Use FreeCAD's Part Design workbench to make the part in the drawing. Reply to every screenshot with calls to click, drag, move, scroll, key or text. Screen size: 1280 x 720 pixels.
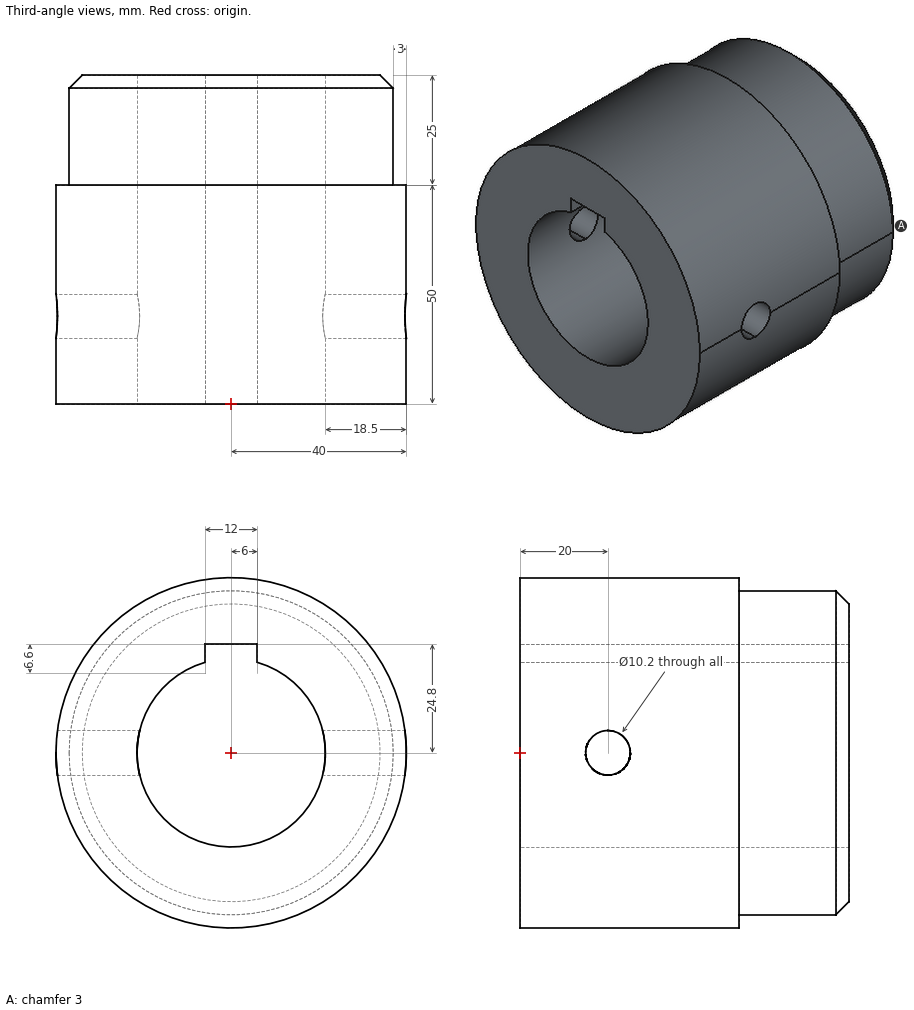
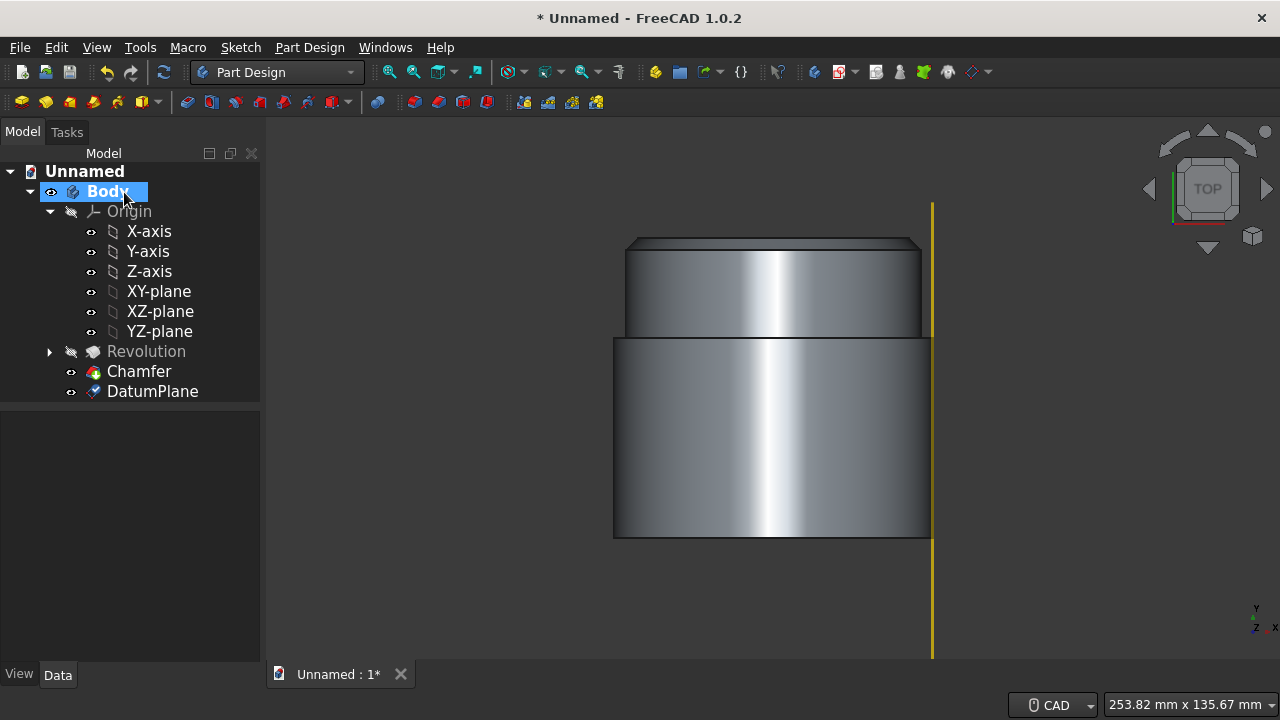
click(116, 392)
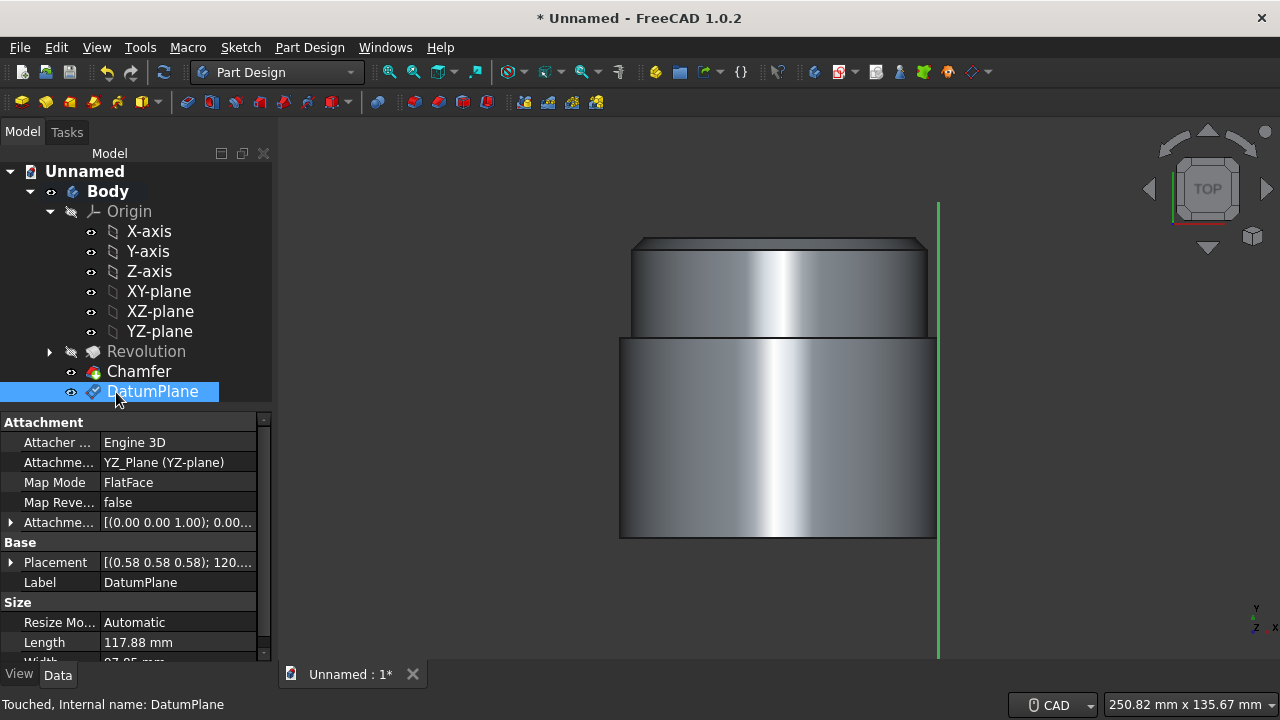
click(840, 72)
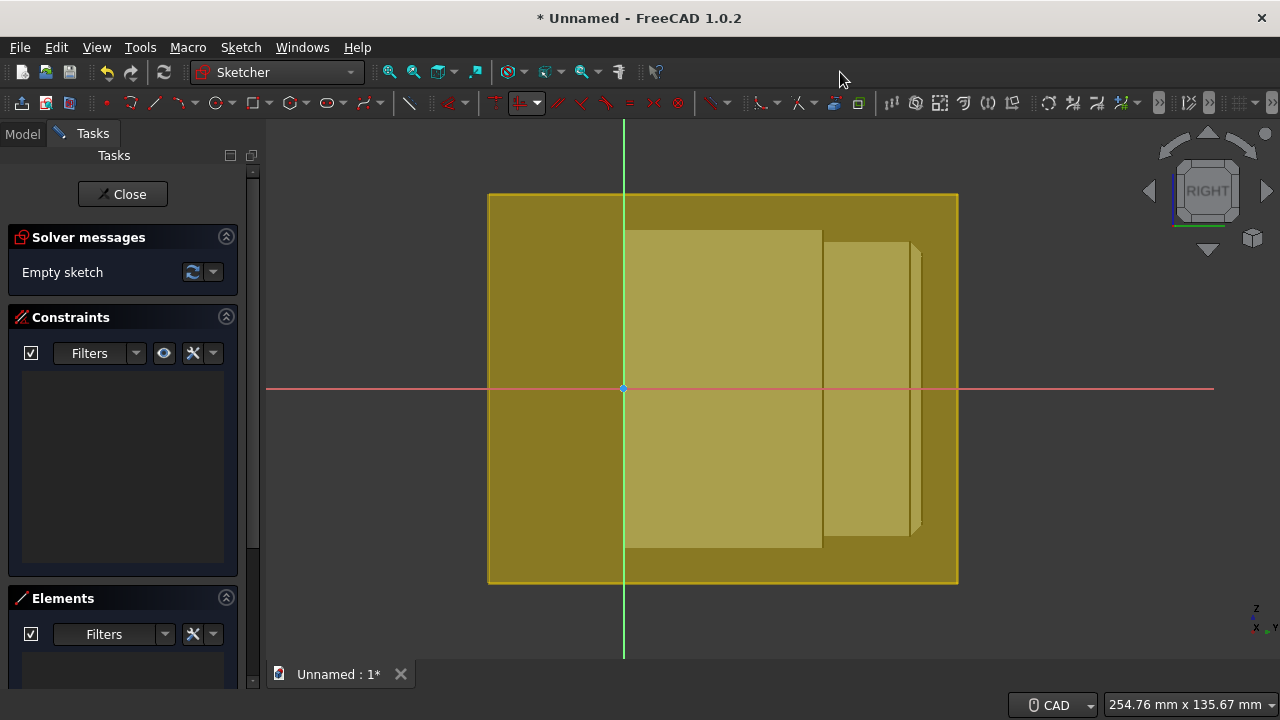
scroll(668, 389, up, 9)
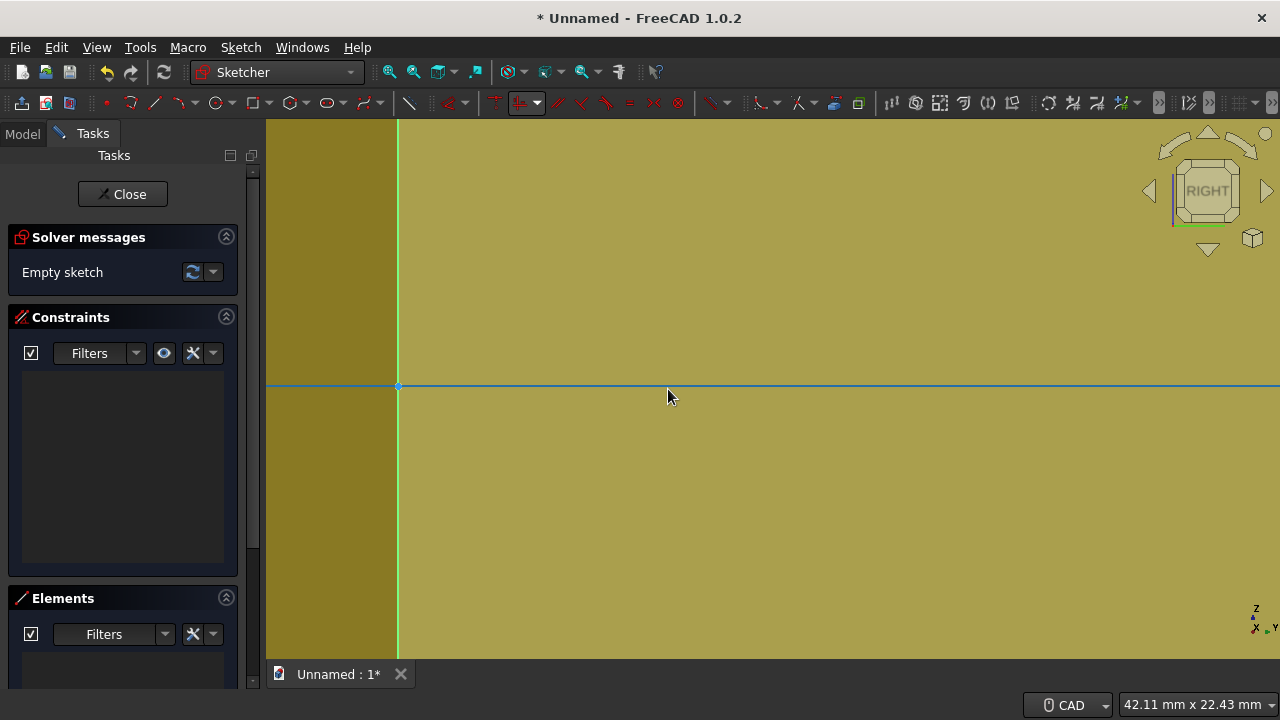
key(g)
key(c)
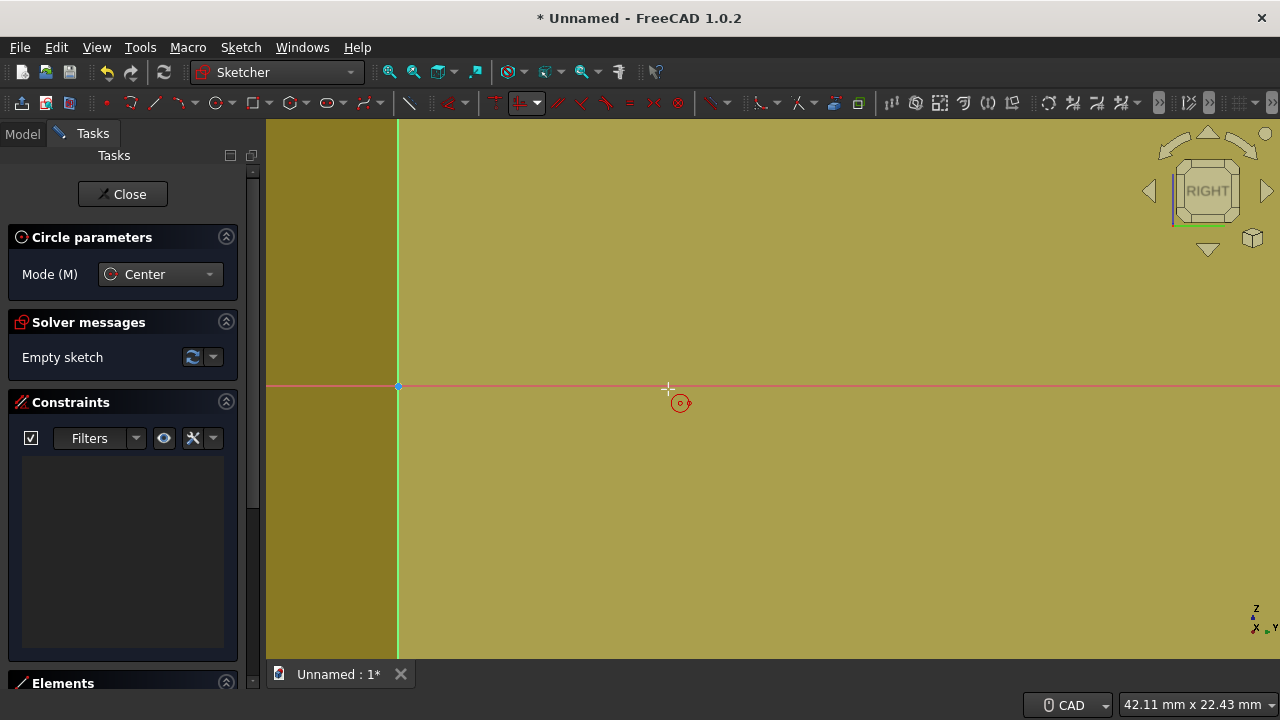
click(880, 386)
move(967, 300)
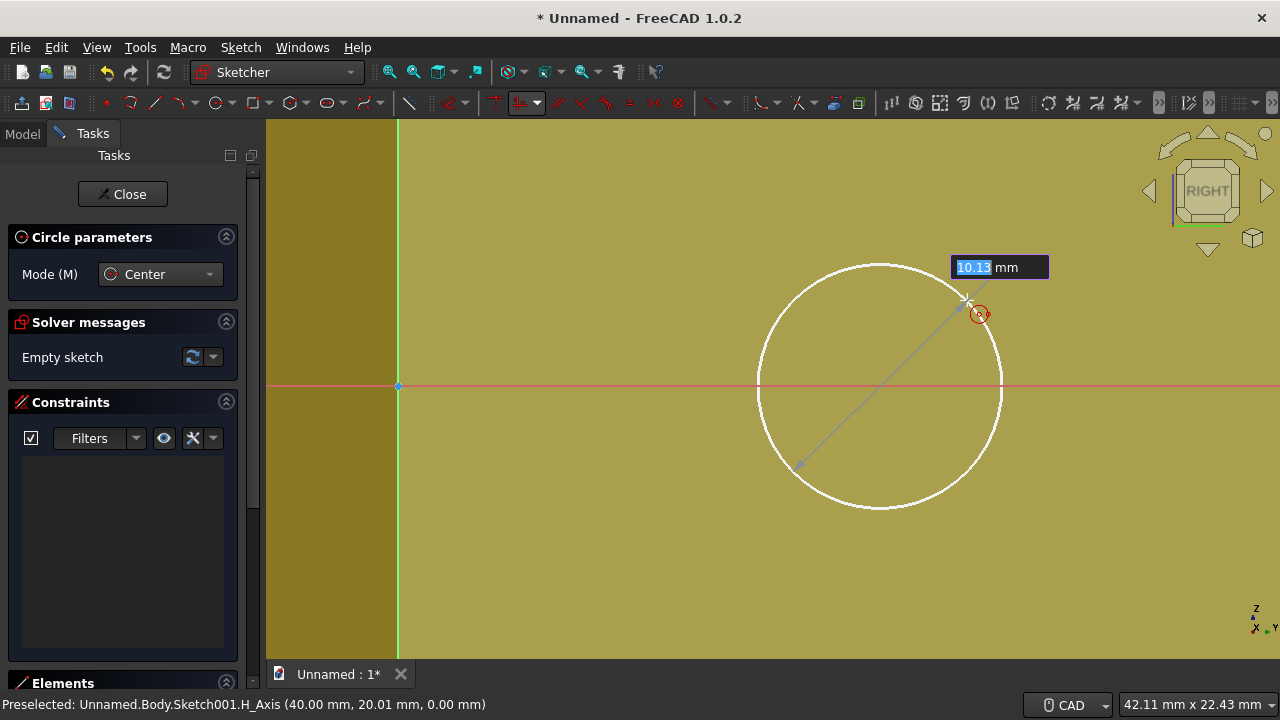
text(10.2)
key(Return)
key(Escape)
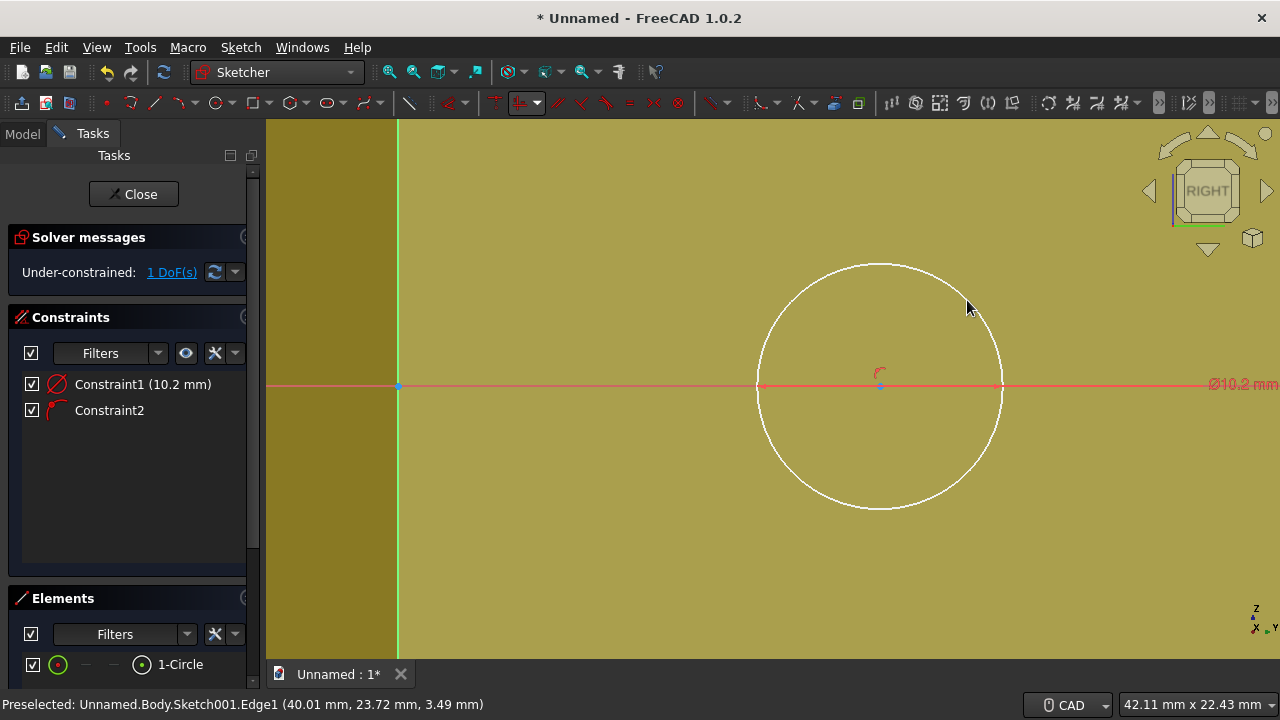
click(448, 104)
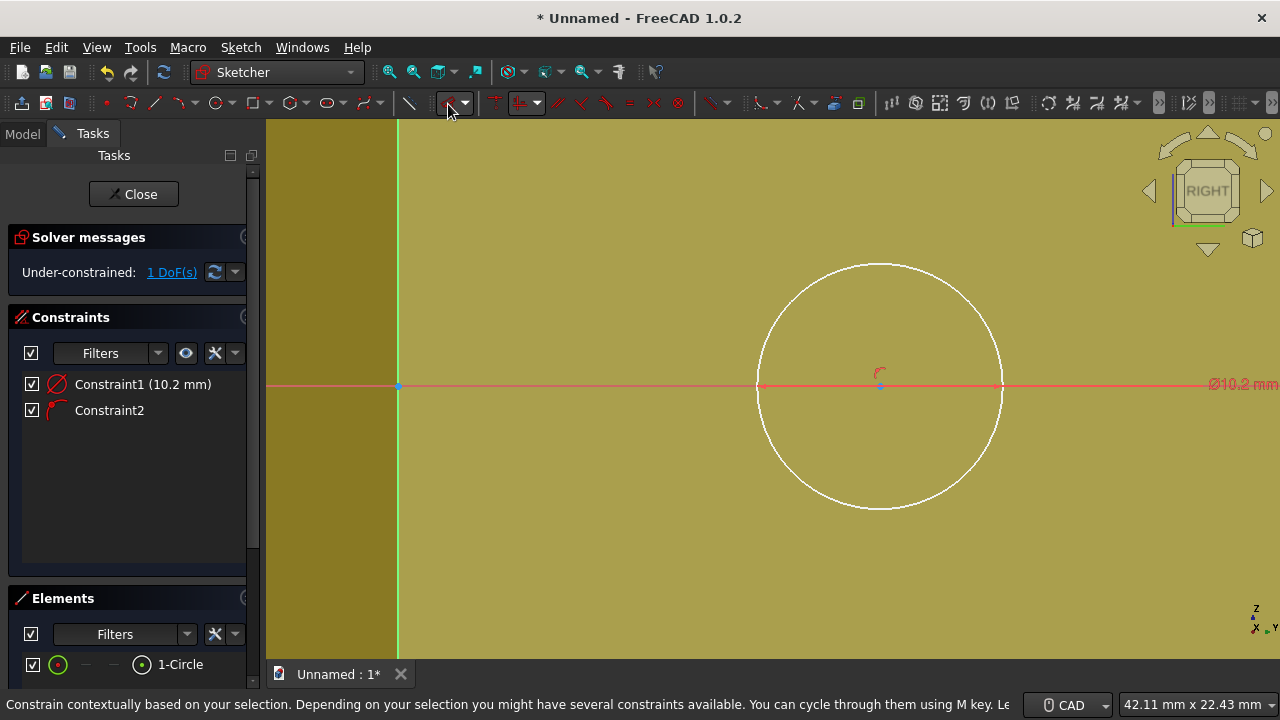
click(880, 386)
click(639, 420)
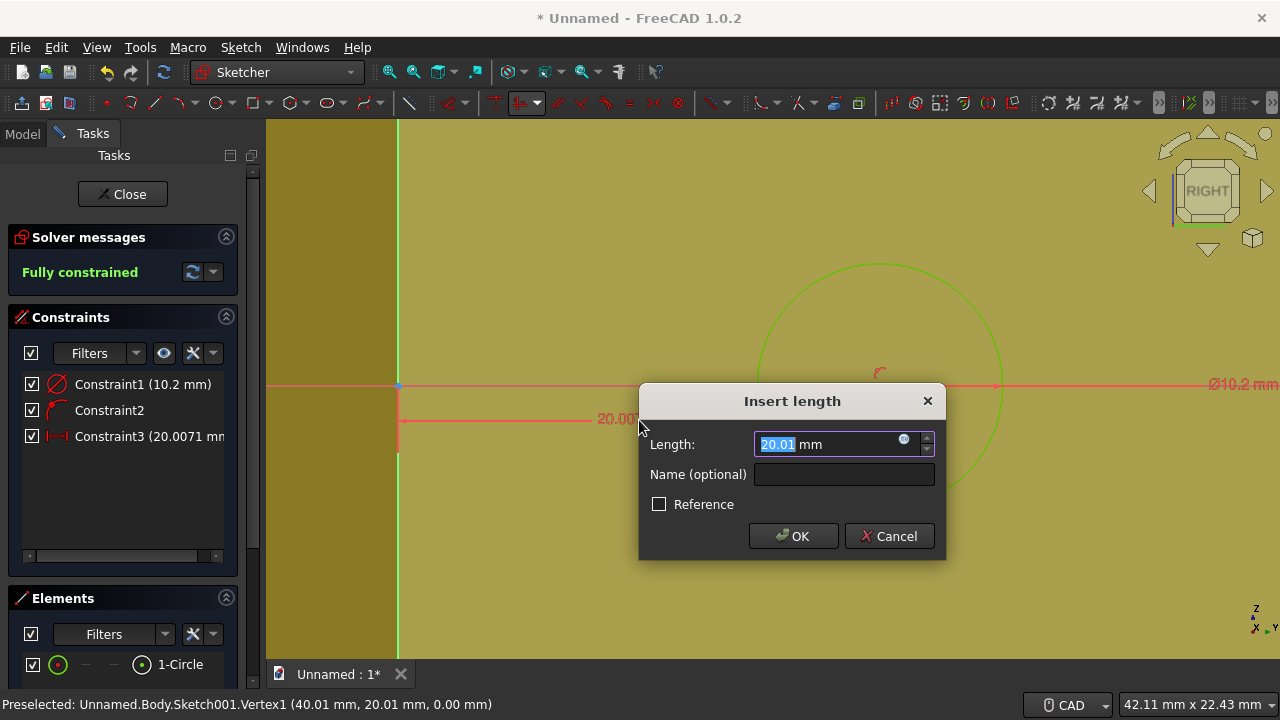
text(20)
key(Return)
key(Escape)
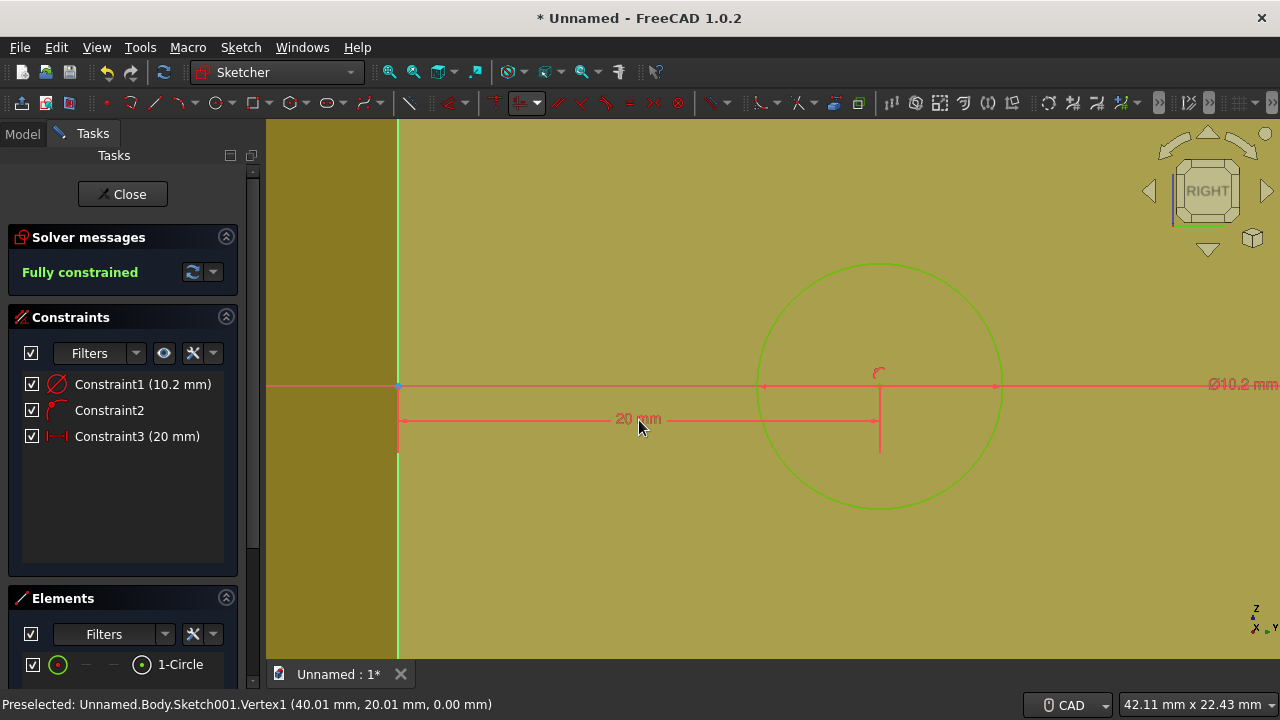
click(123, 194)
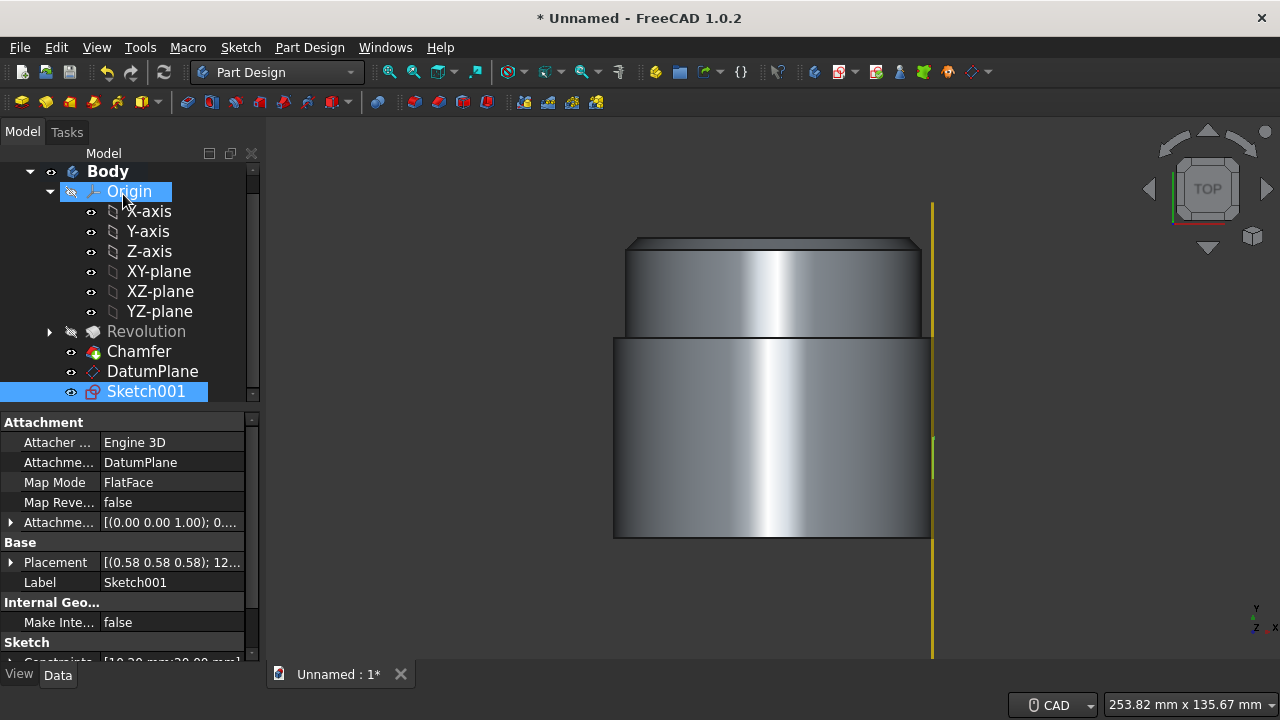
click(212, 102)